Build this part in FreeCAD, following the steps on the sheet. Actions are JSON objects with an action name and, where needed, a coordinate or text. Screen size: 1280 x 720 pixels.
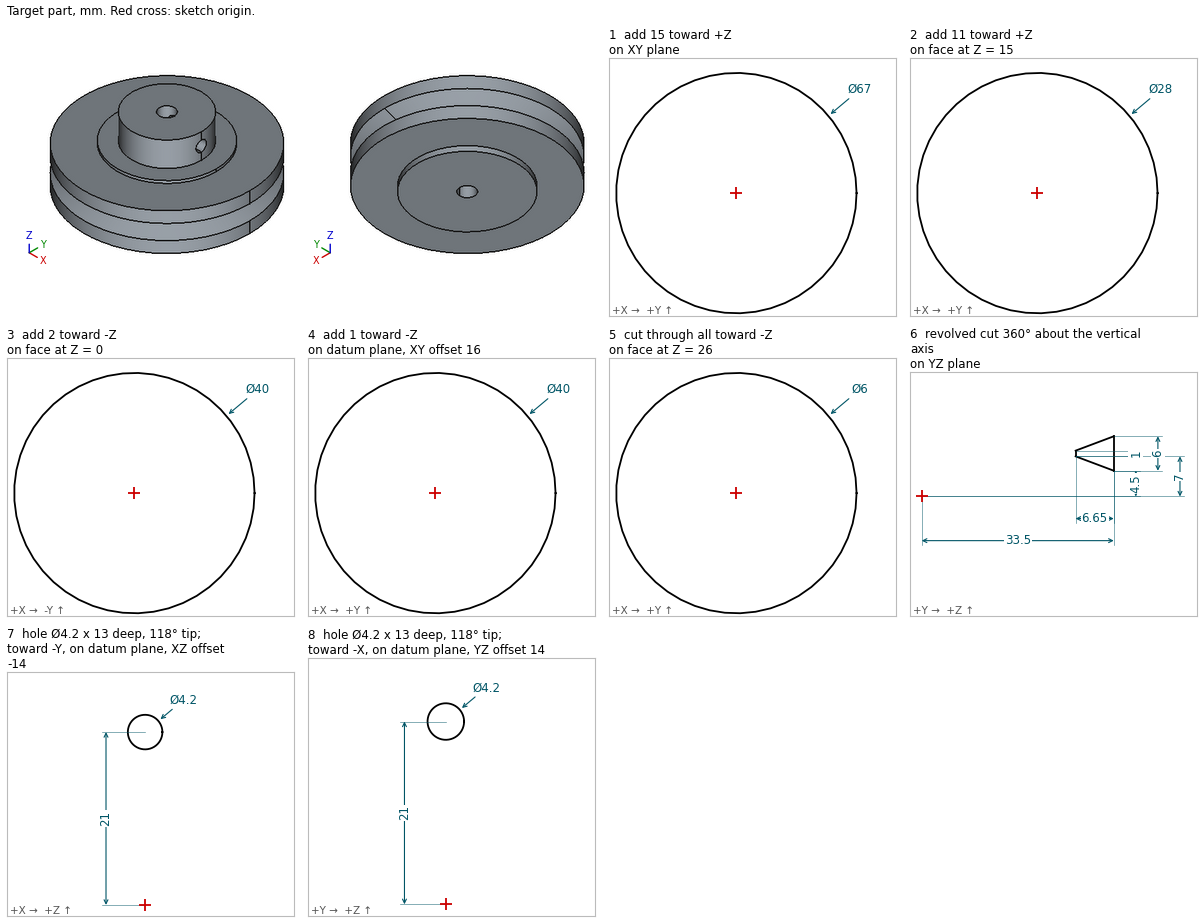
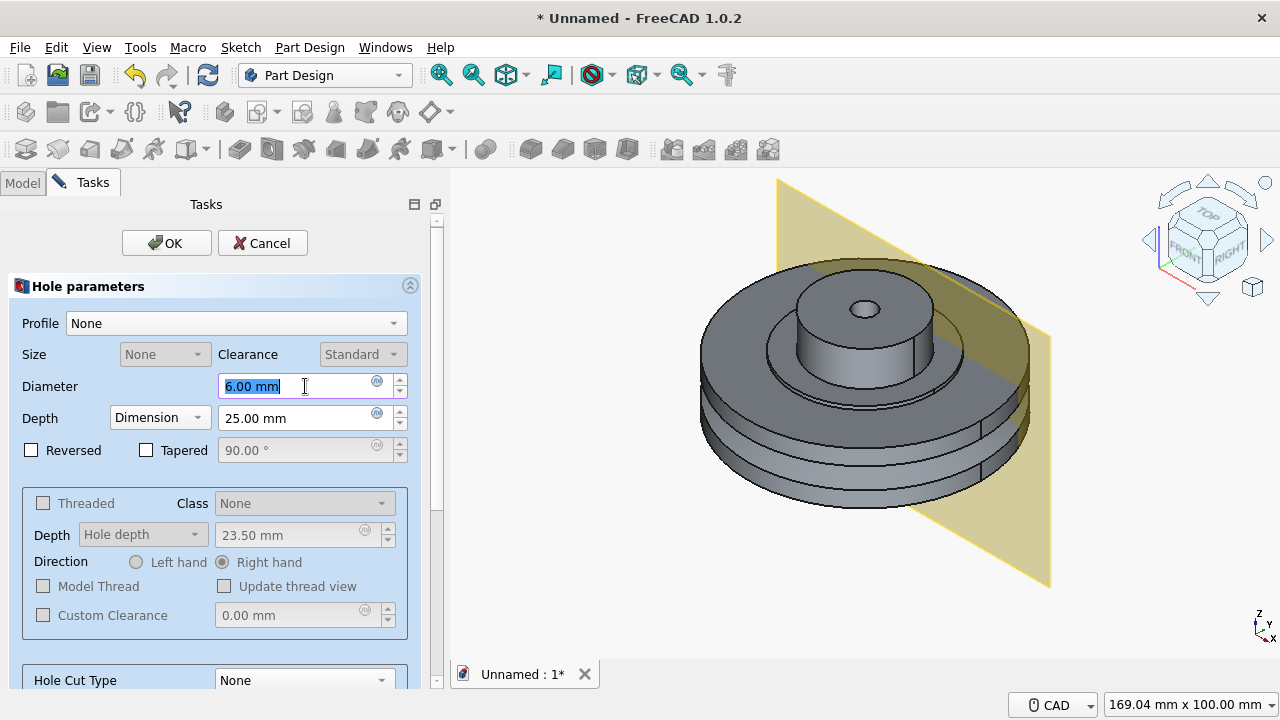
{"action": "type", "text": "4.2"}
{"action": "key", "text": "Tab"}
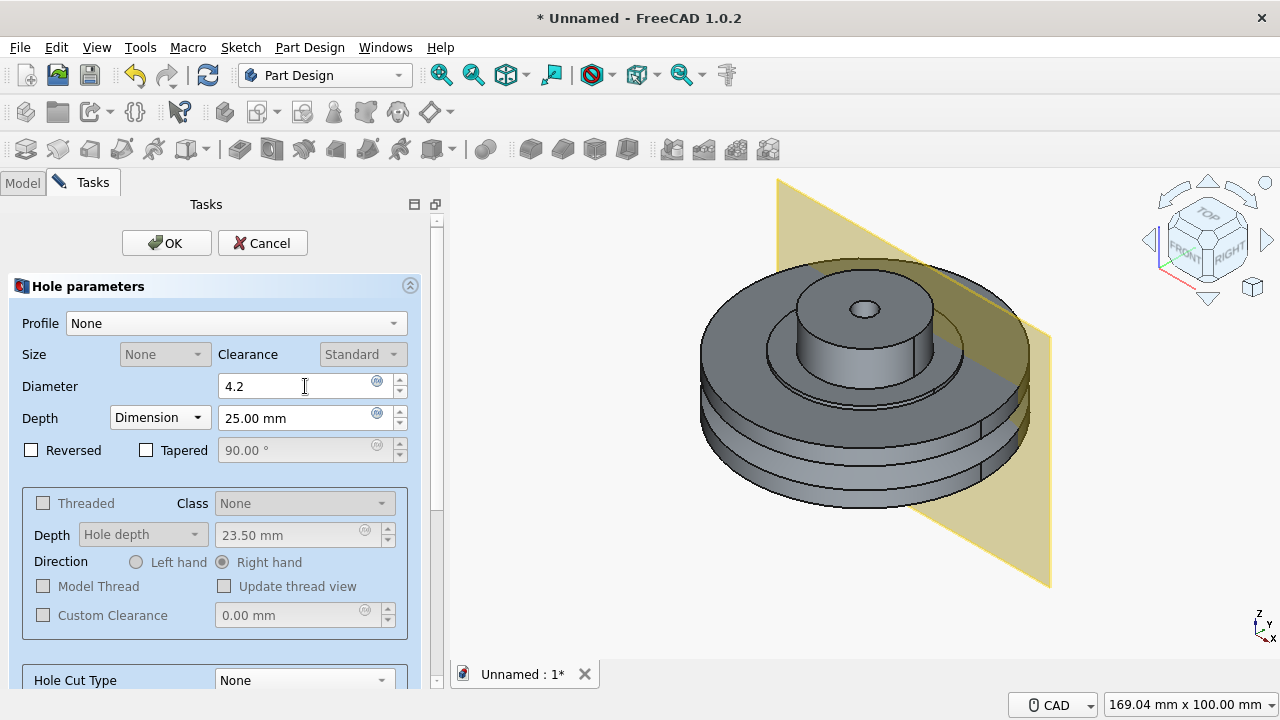
{"action": "triple_click", "coordinate": [305, 418]}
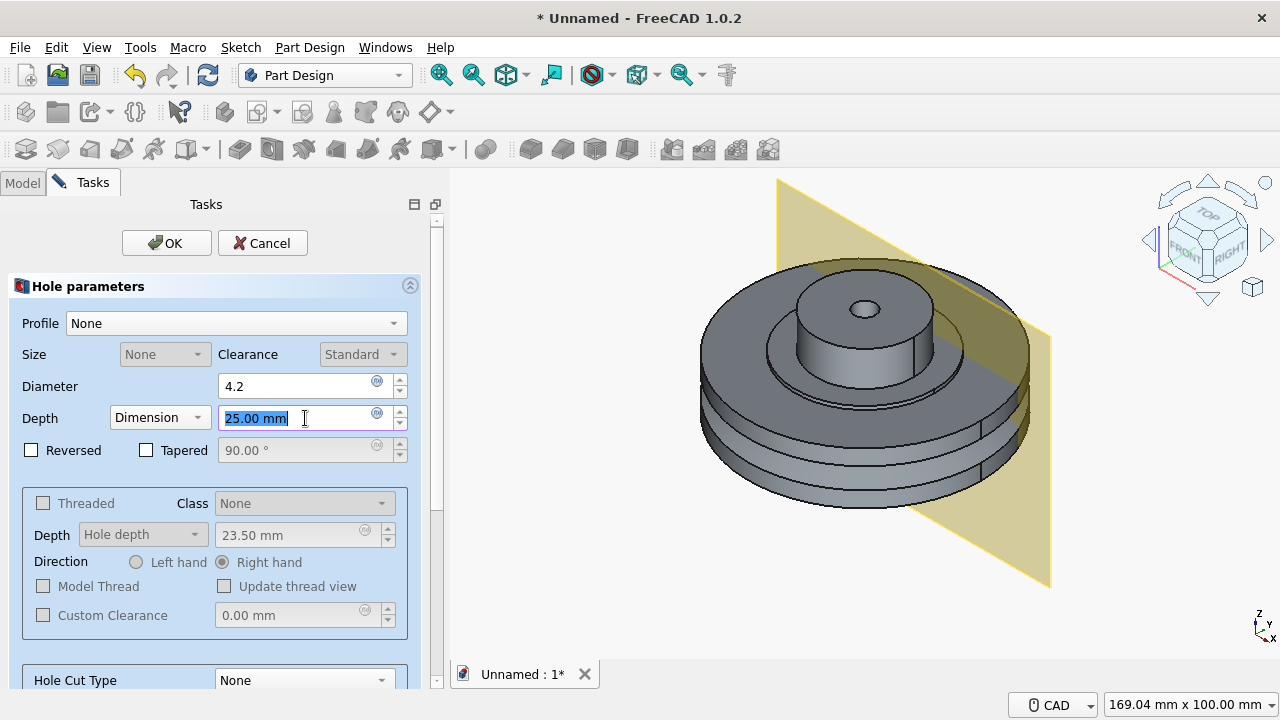
{"action": "type", "text": "13"}
{"action": "key", "text": "Tab"}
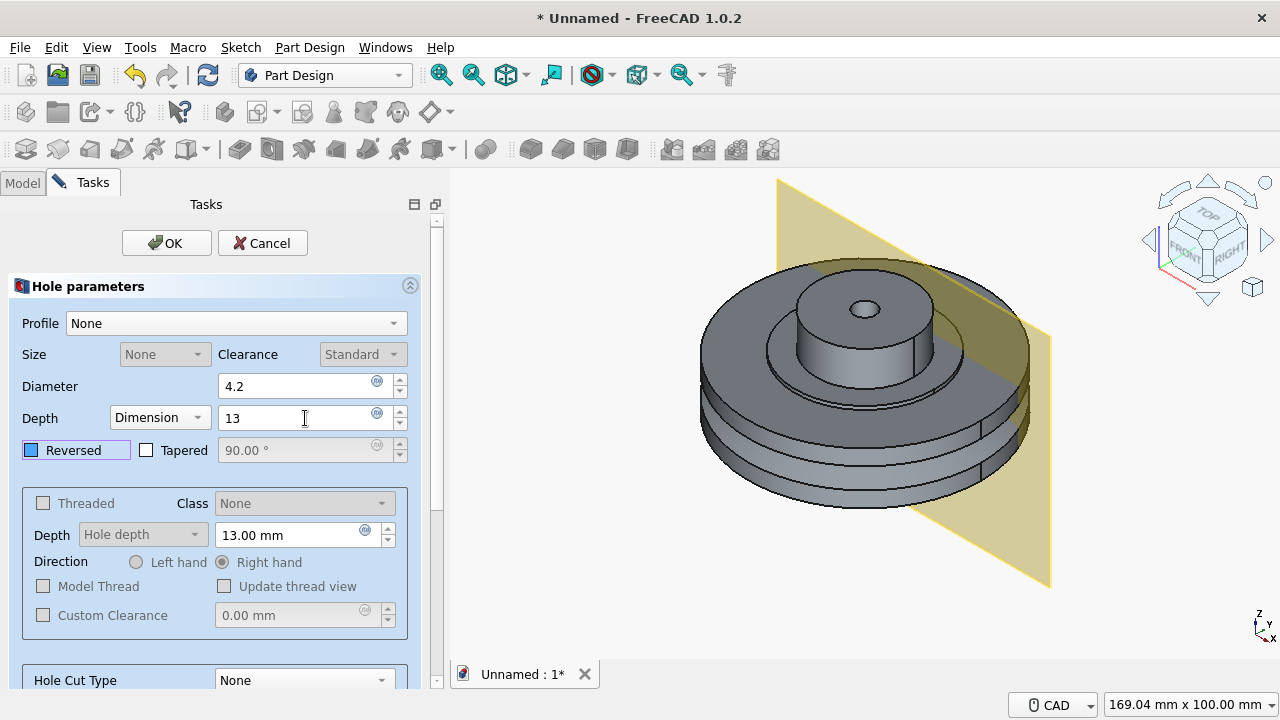
{"action": "left_click", "coordinate": [30, 450]}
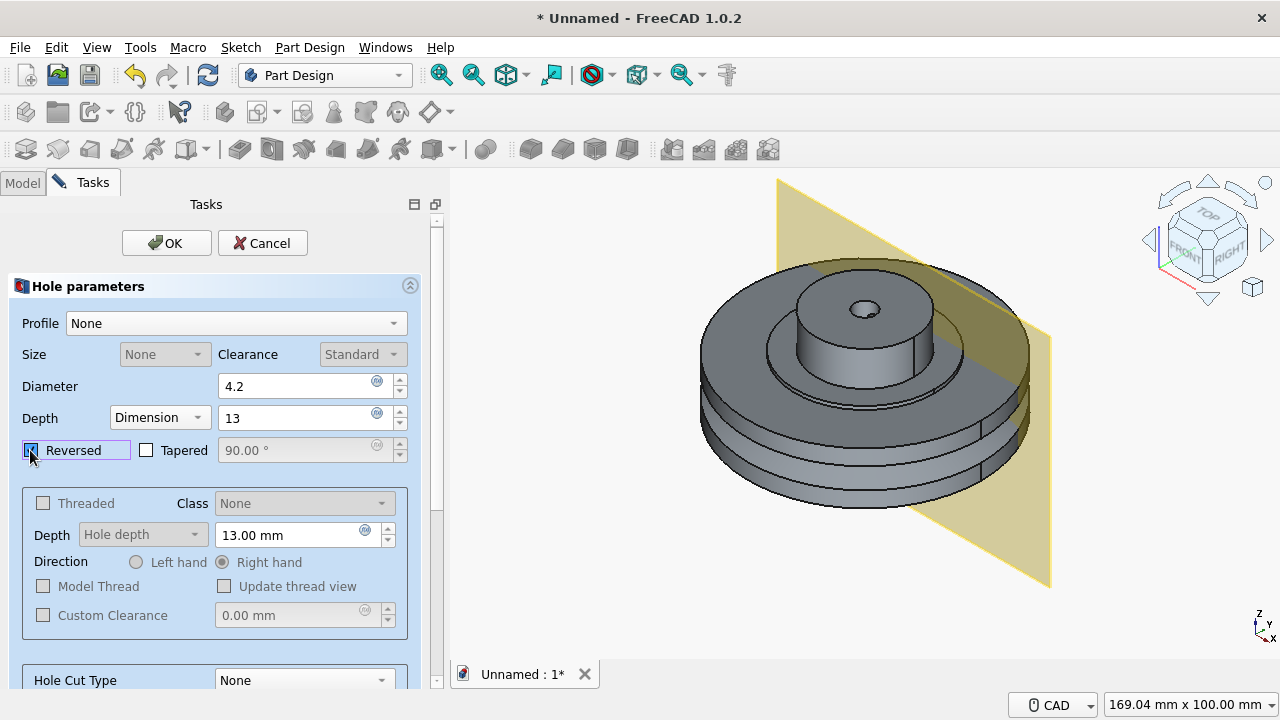
{"action": "left_click", "coordinate": [167, 243]}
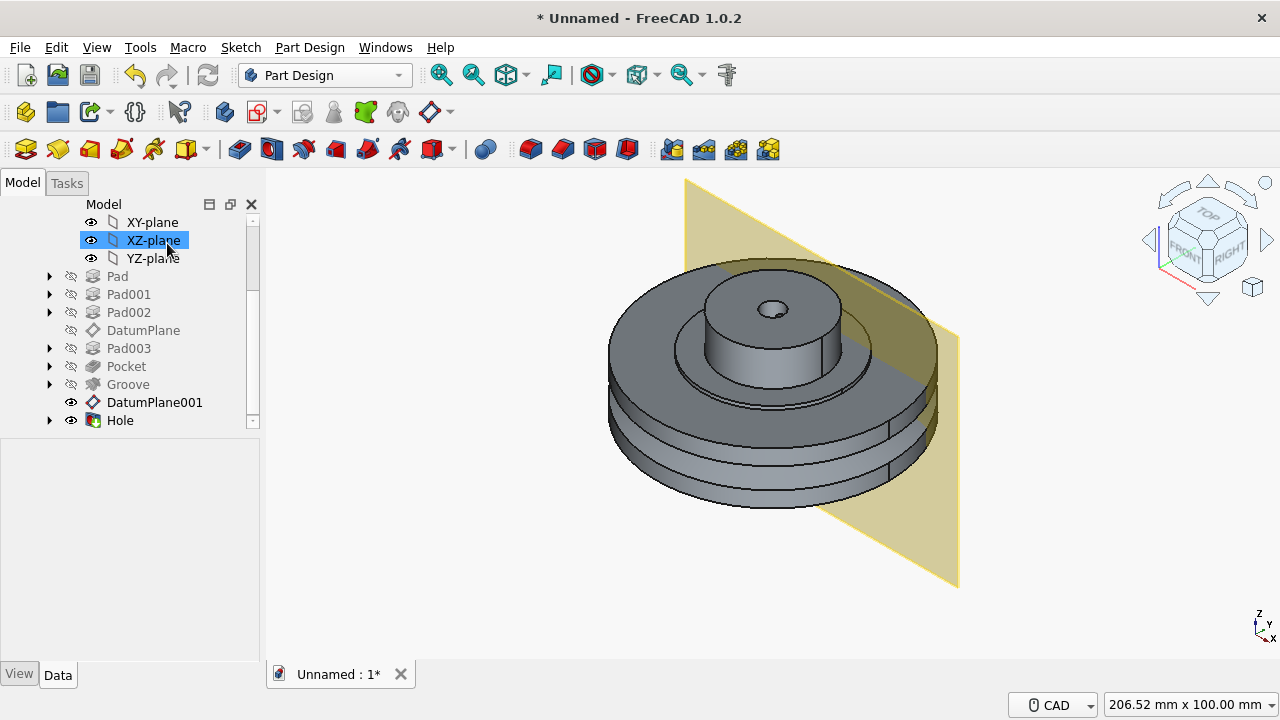
{"action": "left_click", "coordinate": [116, 402]}
{"action": "key", "text": "space"}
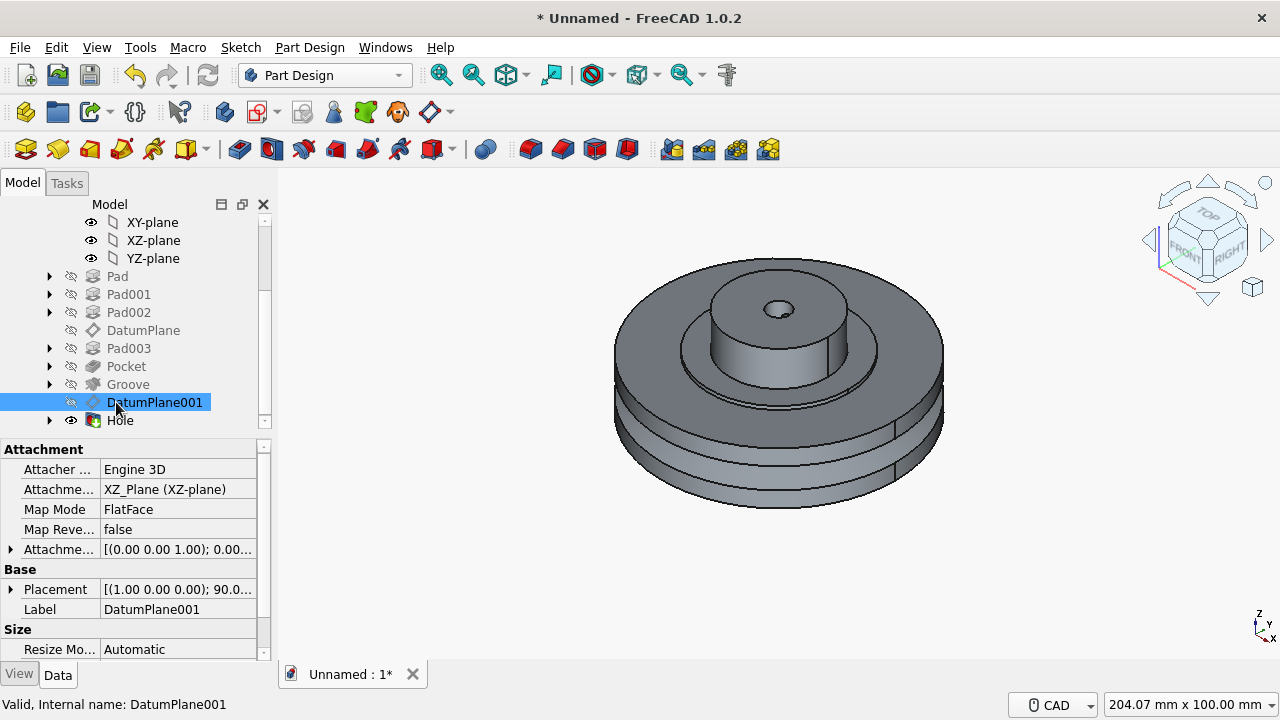
{"action": "scroll", "coordinate": [160, 326], "scroll_direction": "down", "scroll_amount": 3}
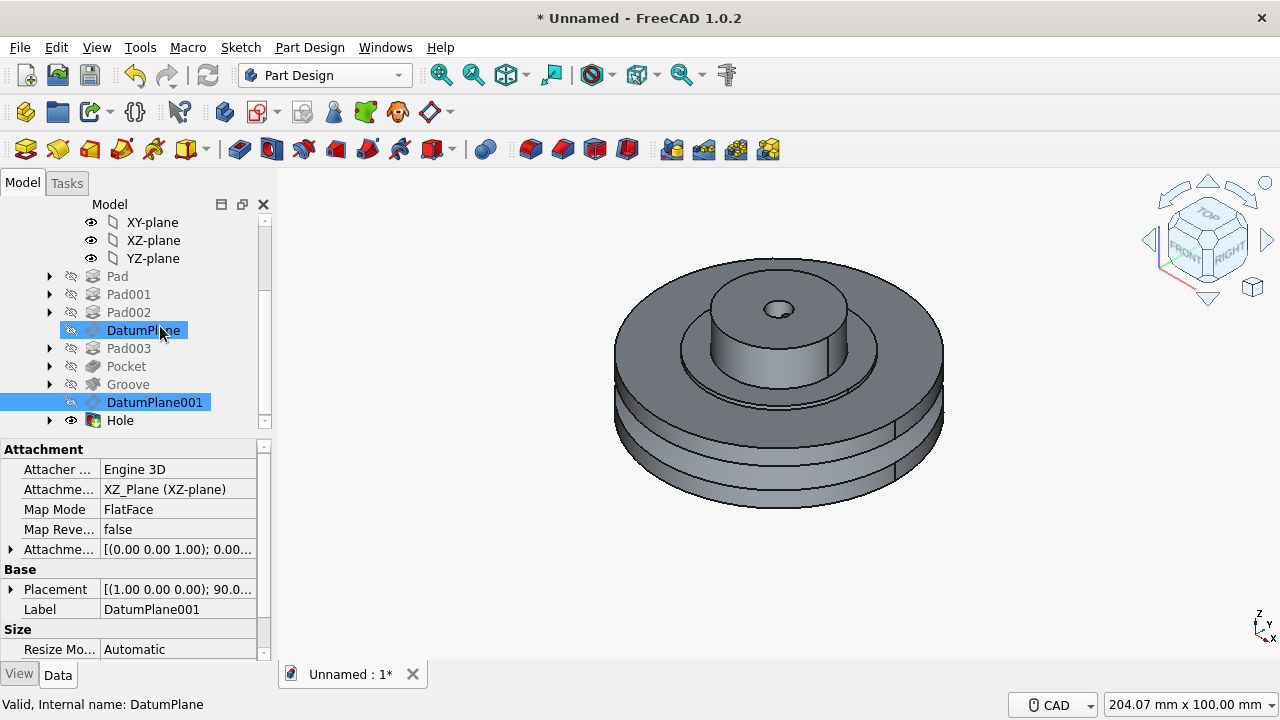
{"action": "scroll", "coordinate": [160, 326], "scroll_direction": "up", "scroll_amount": 15}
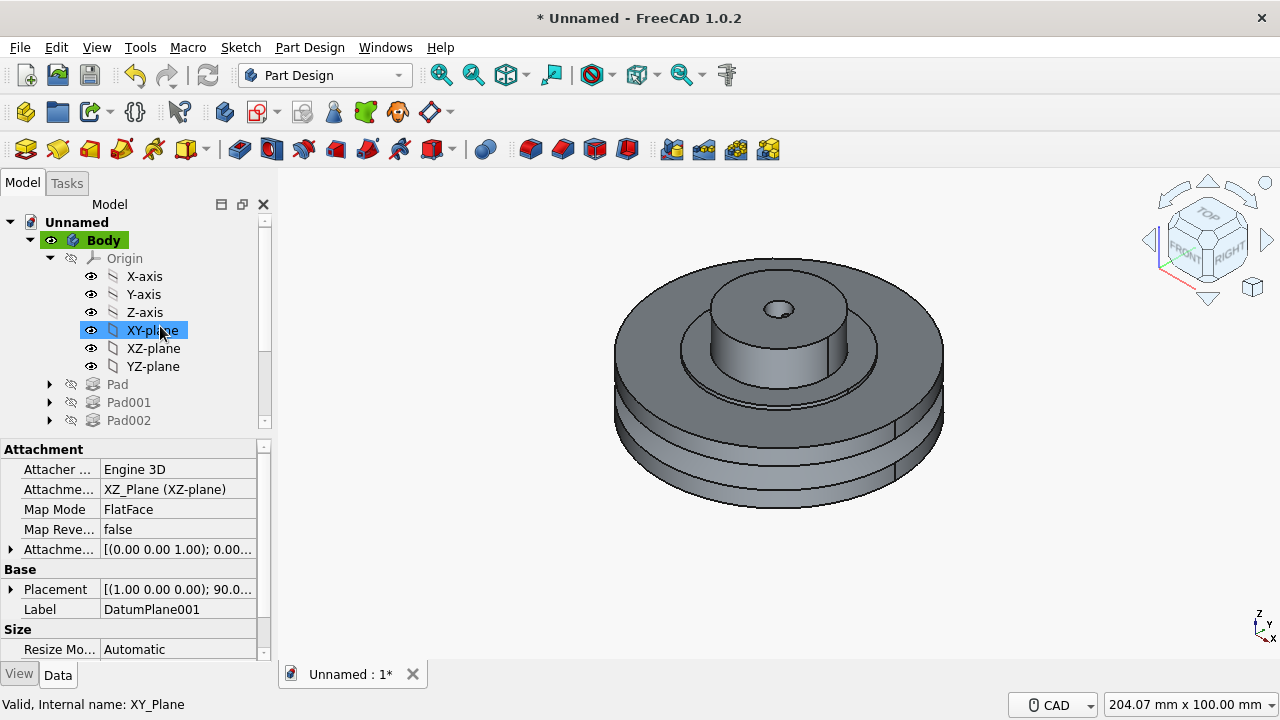
{"action": "left_click", "coordinate": [136, 366]}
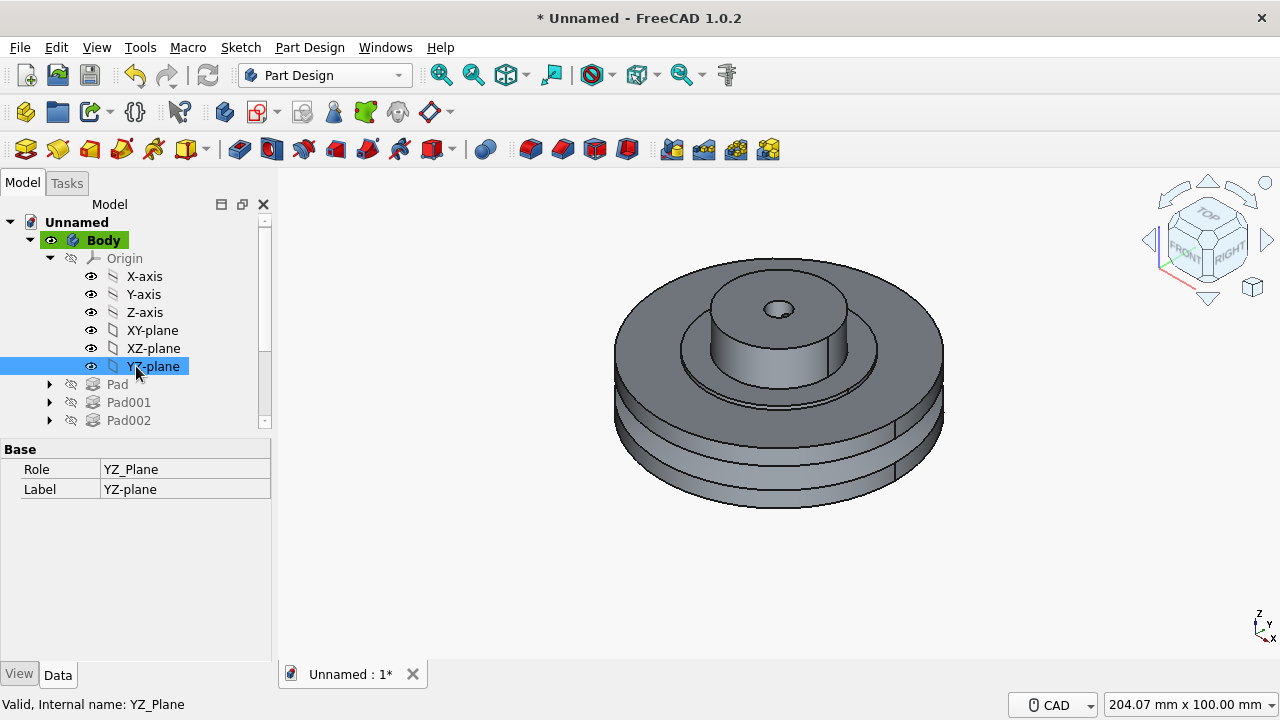
{"action": "left_click", "coordinate": [430, 112]}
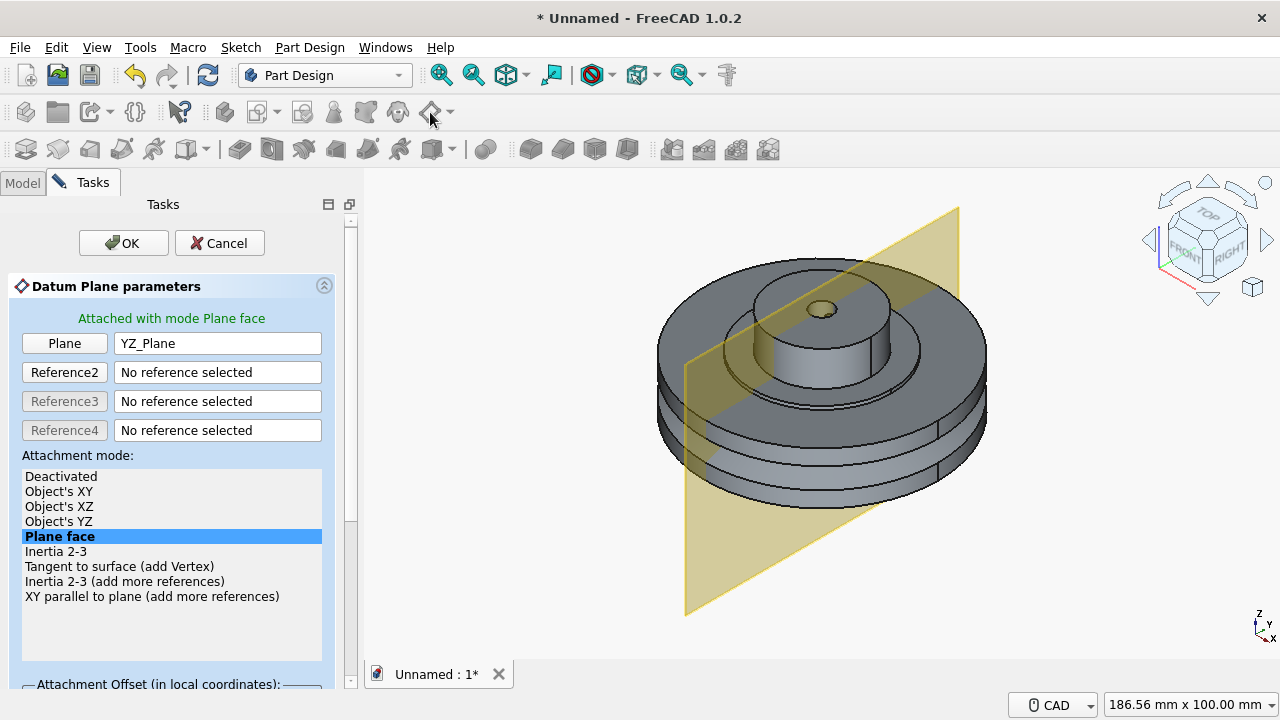
{"action": "scroll", "coordinate": [351, 451], "scroll_direction": "down", "scroll_amount": 3}